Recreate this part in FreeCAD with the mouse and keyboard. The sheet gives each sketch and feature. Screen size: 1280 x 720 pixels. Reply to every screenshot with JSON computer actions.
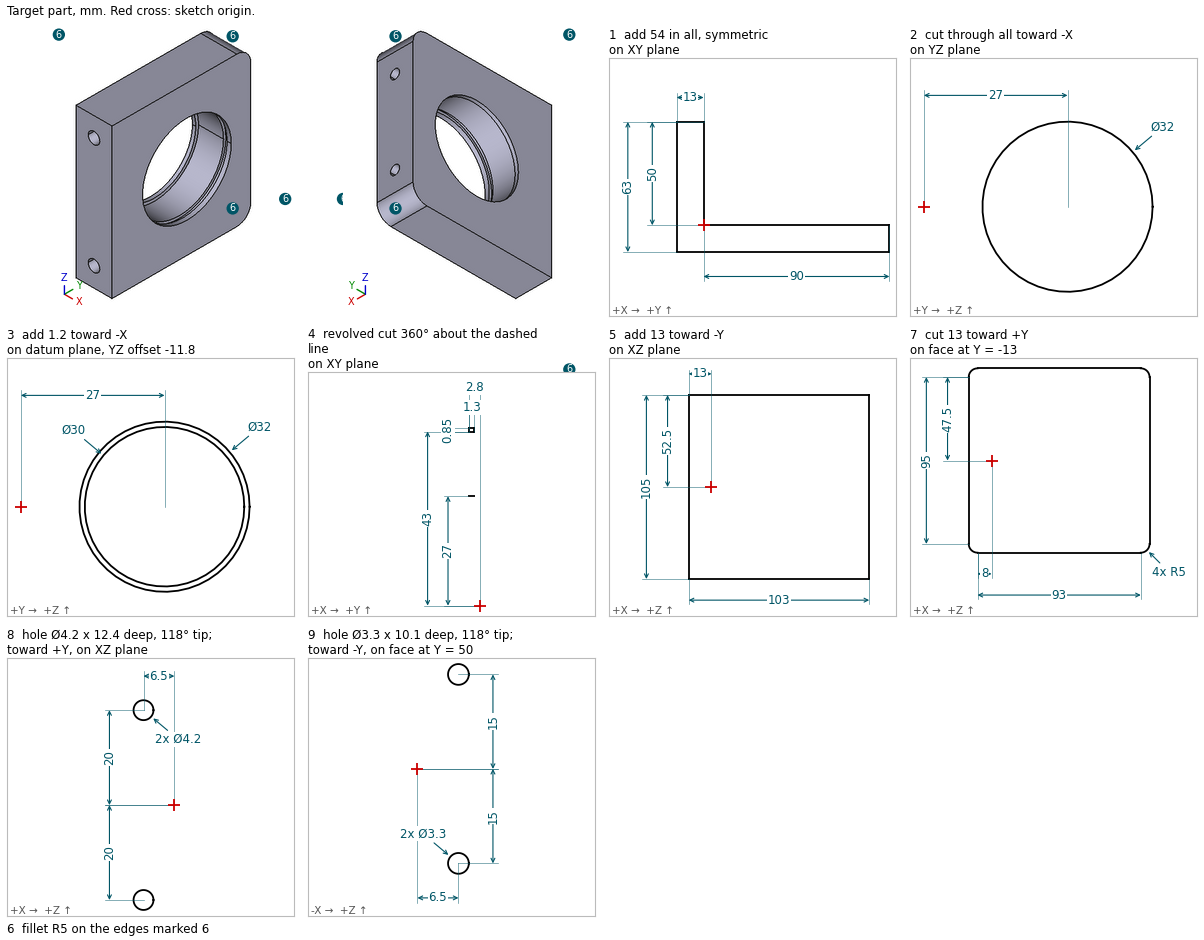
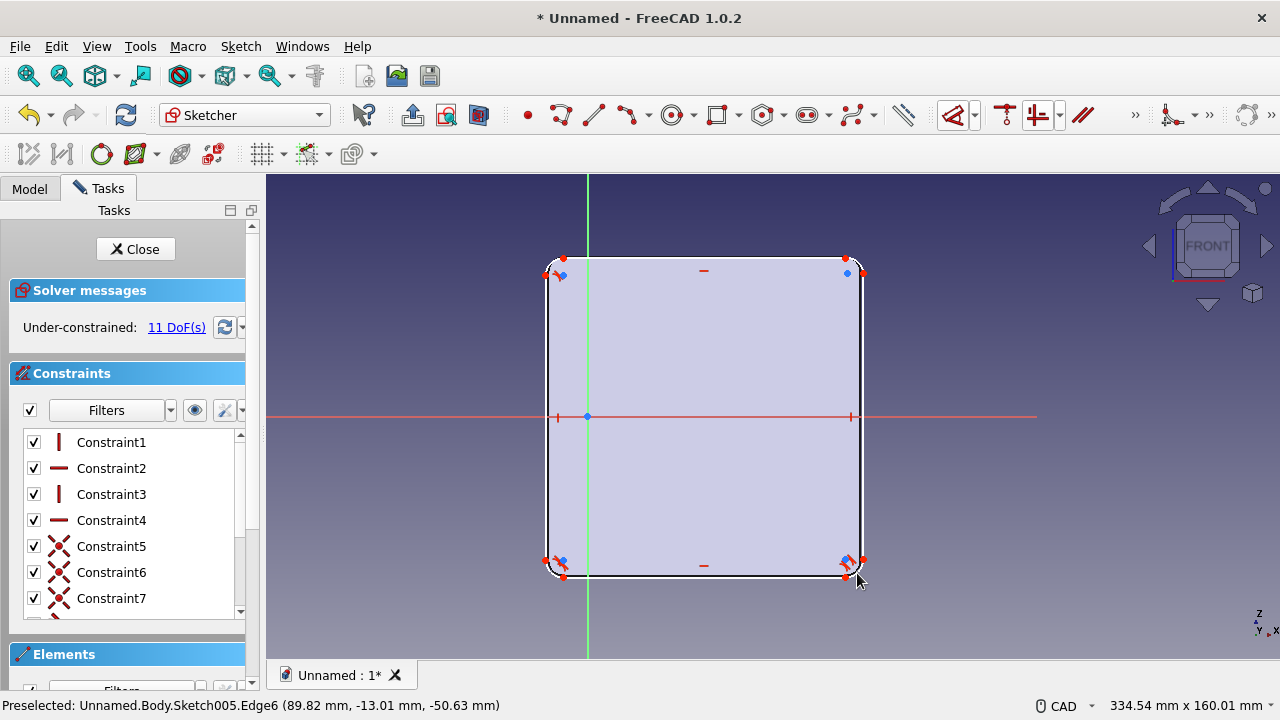
{"action": "left_click", "coordinate": [863, 474]}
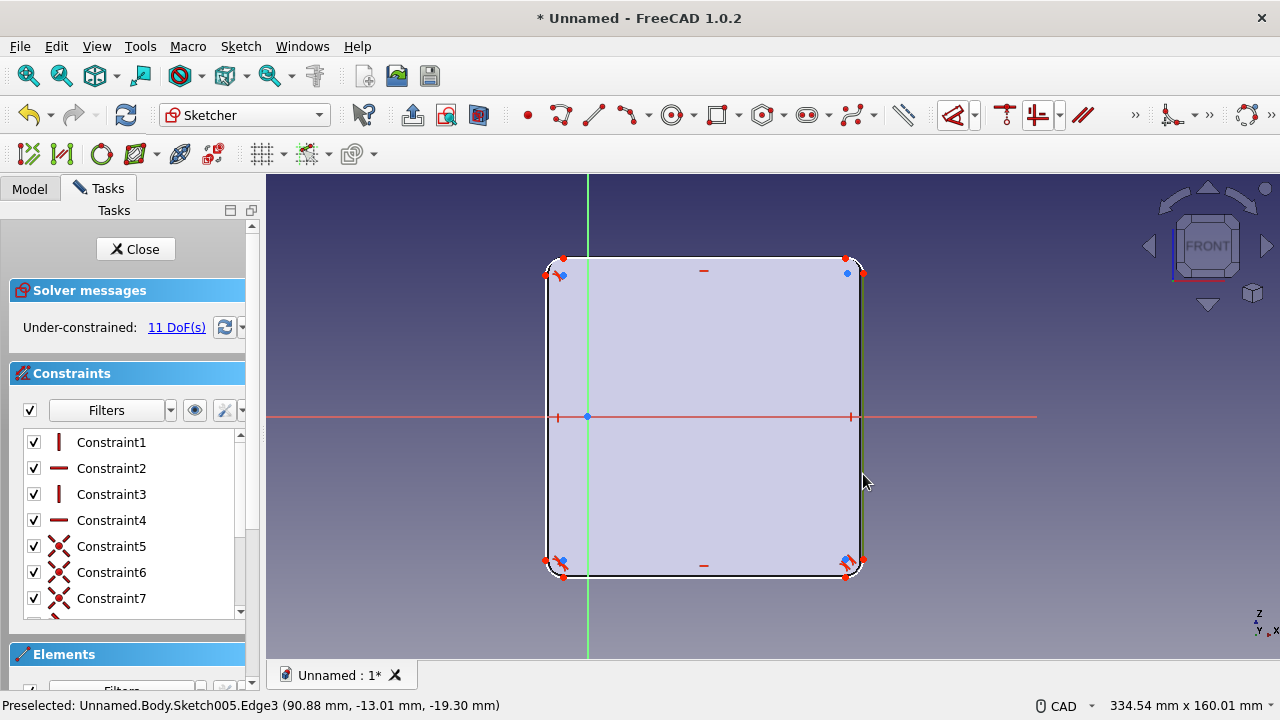
{"action": "left_click", "coordinate": [858, 262]}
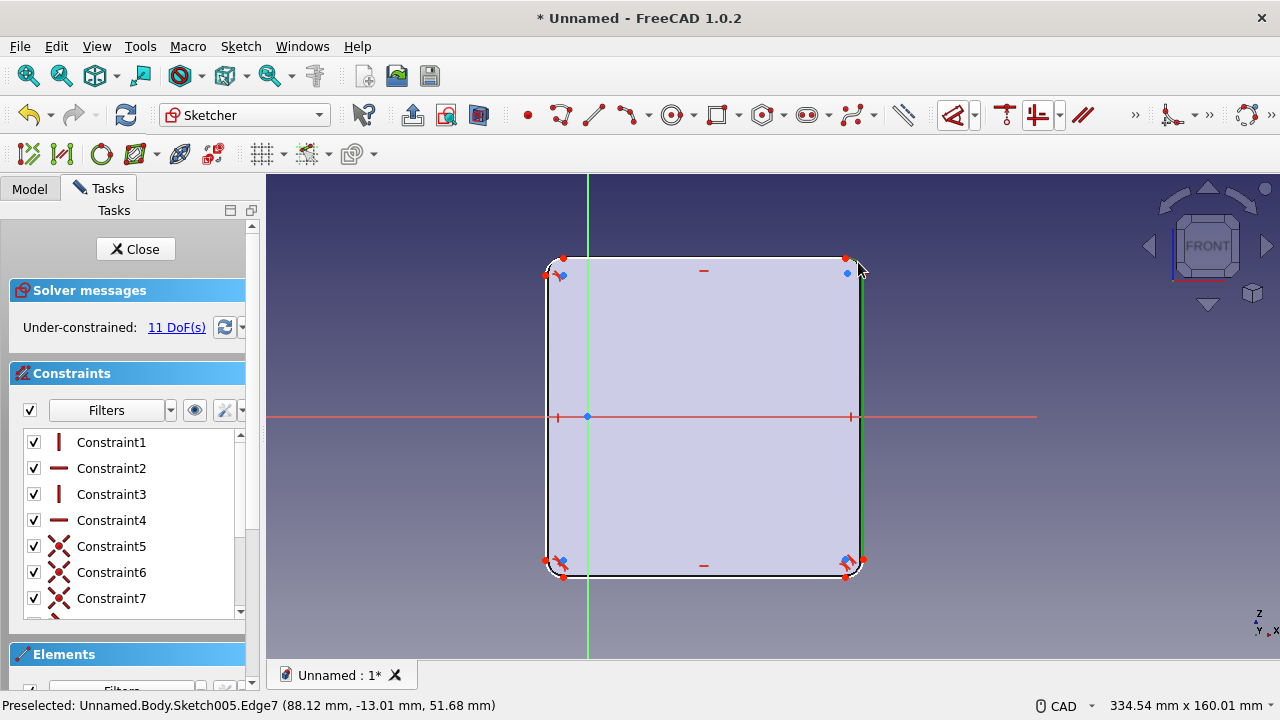
{"action": "key", "text": "t"}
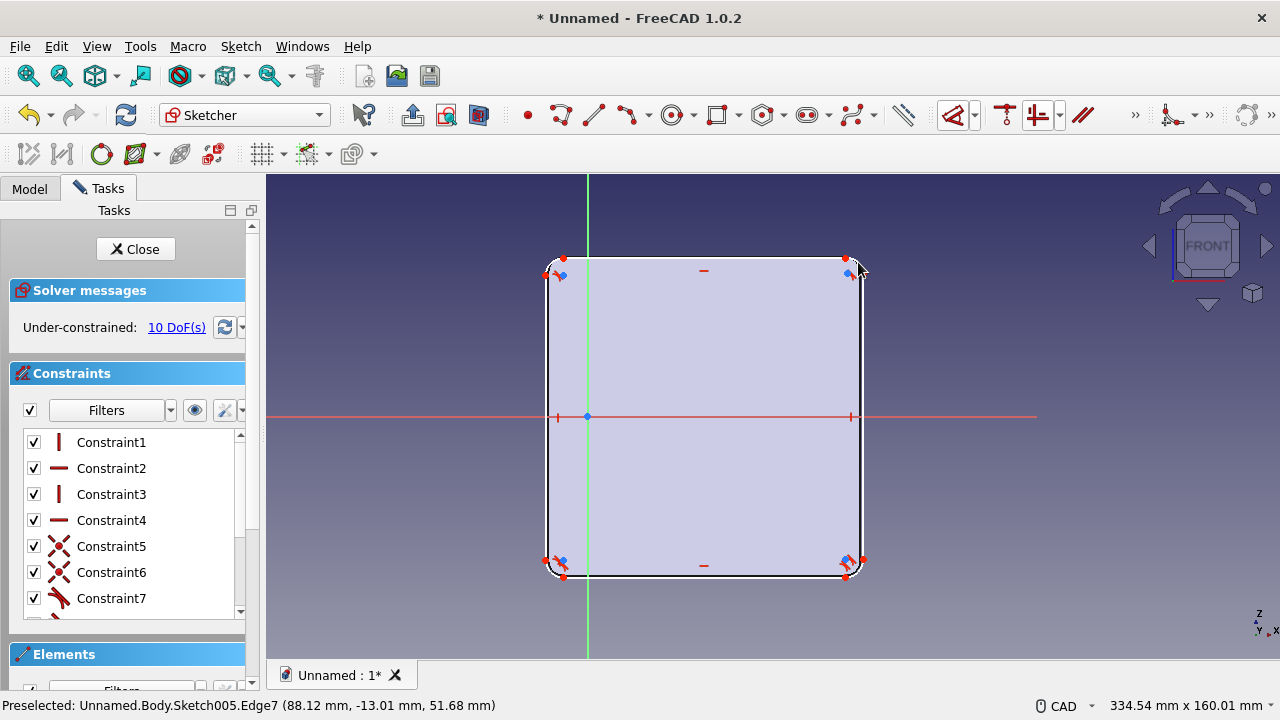
{"action": "left_click", "coordinate": [761, 258]}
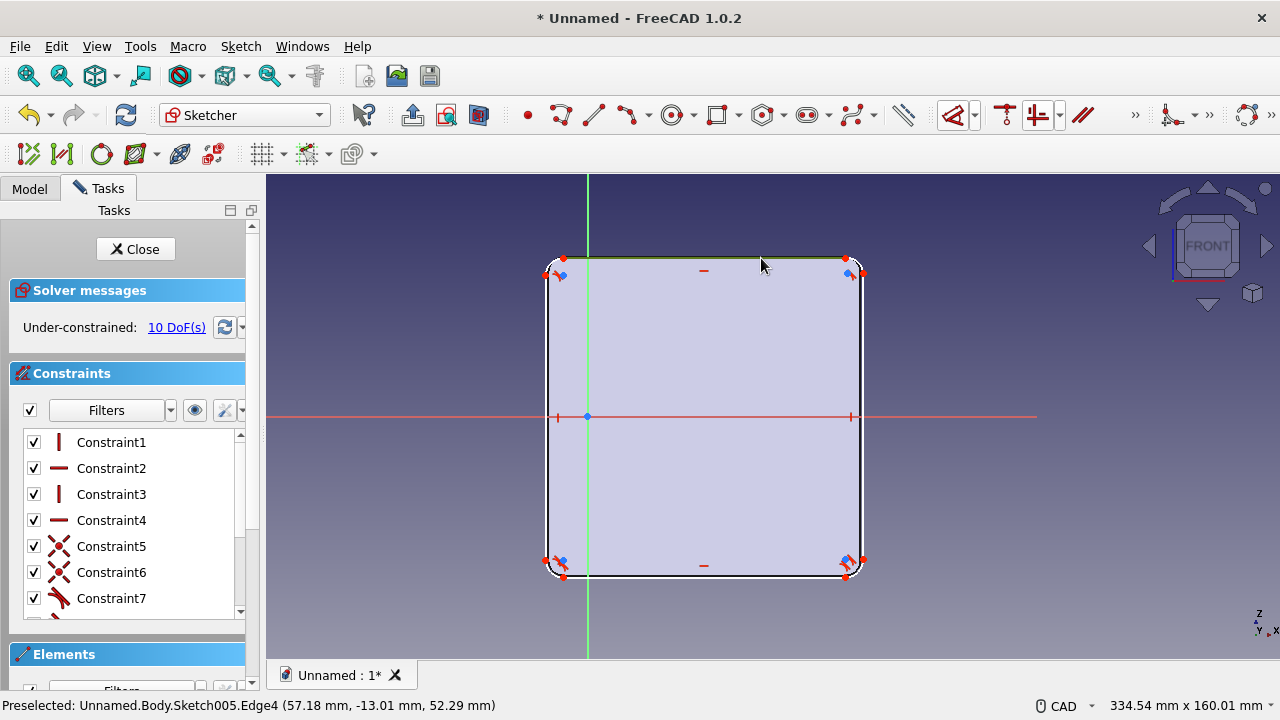
{"action": "left_click", "coordinate": [858, 262]}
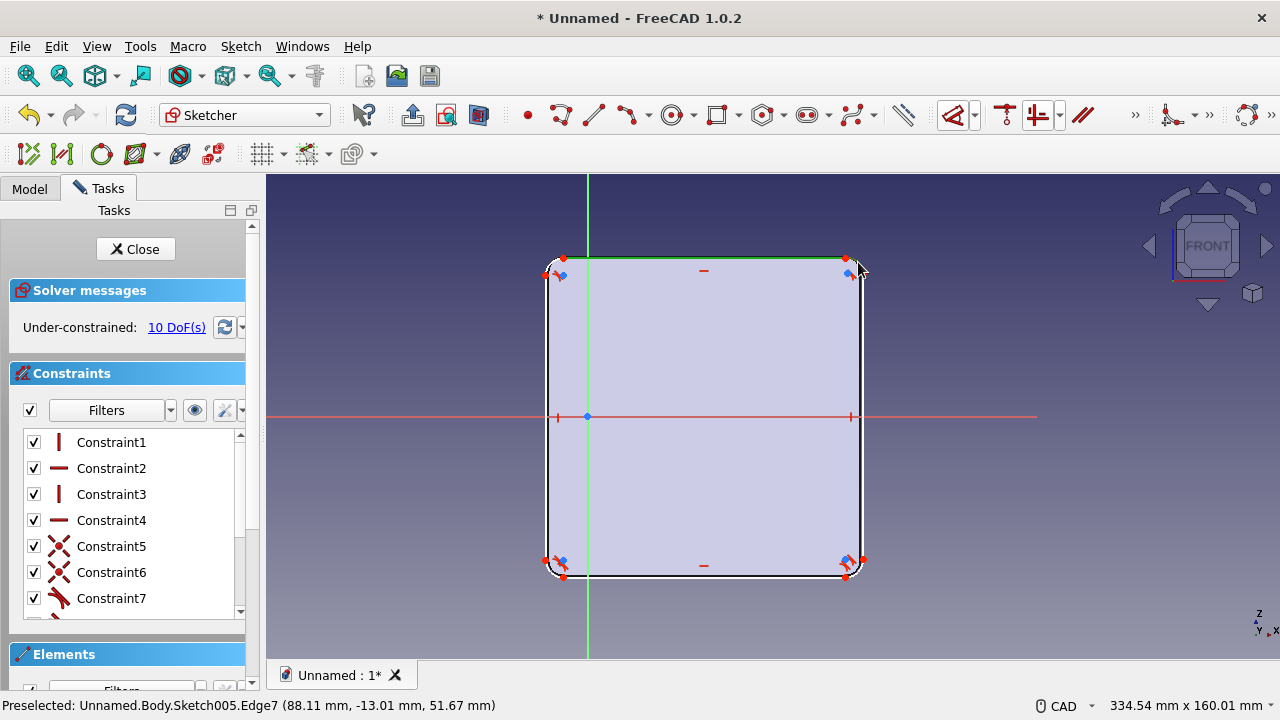
{"action": "key", "text": "t"}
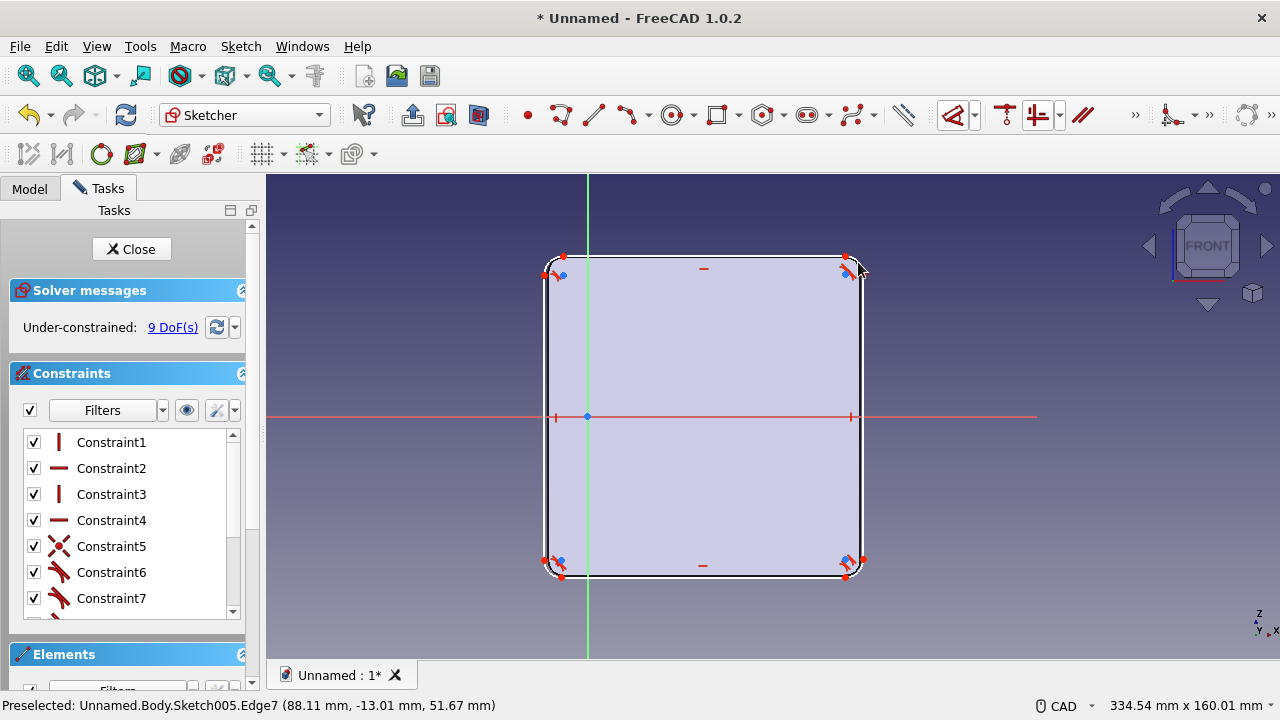
{"action": "left_click", "coordinate": [761, 256]}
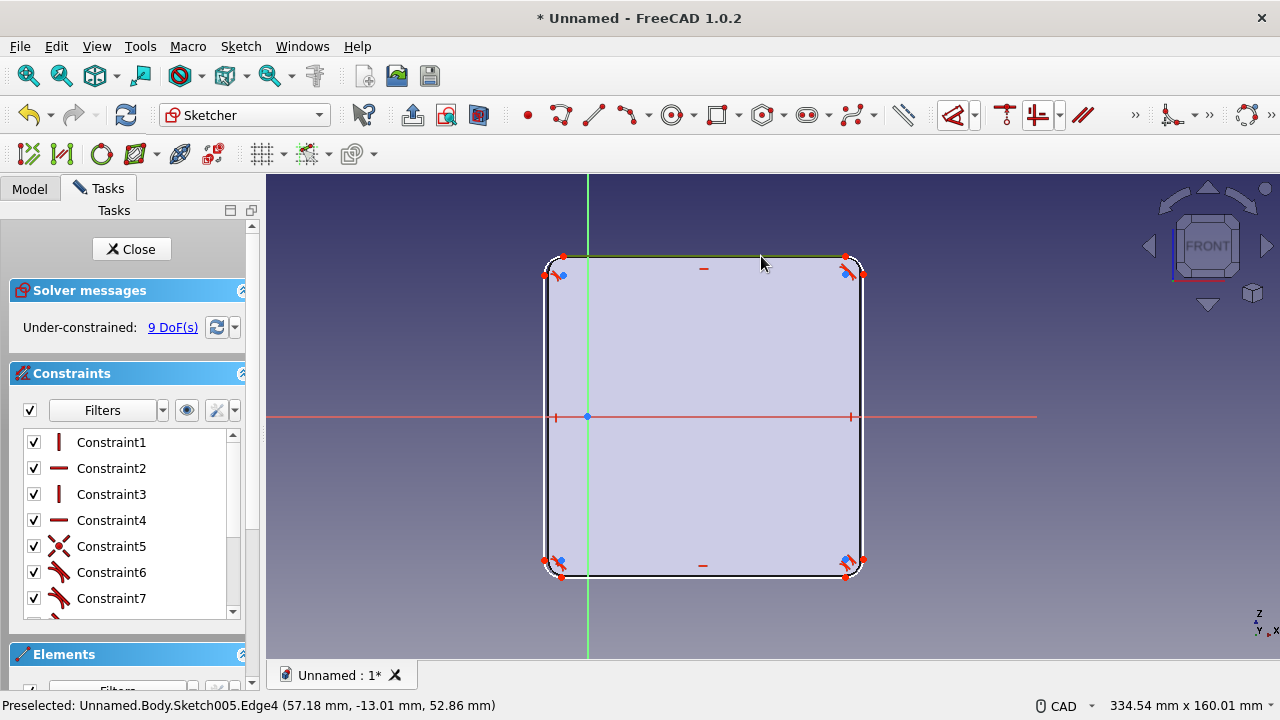
{"action": "scroll", "coordinate": [555, 258], "scroll_direction": "up", "scroll_amount": 3}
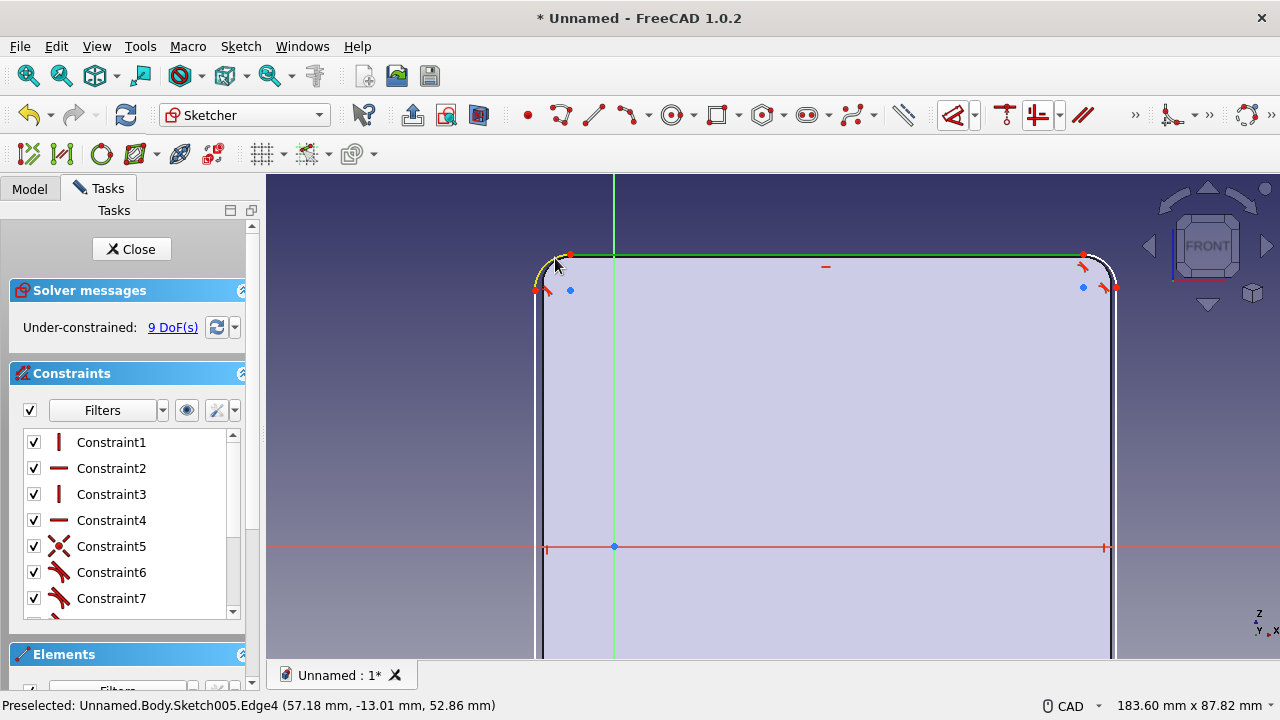
{"action": "left_click", "coordinate": [554, 259]}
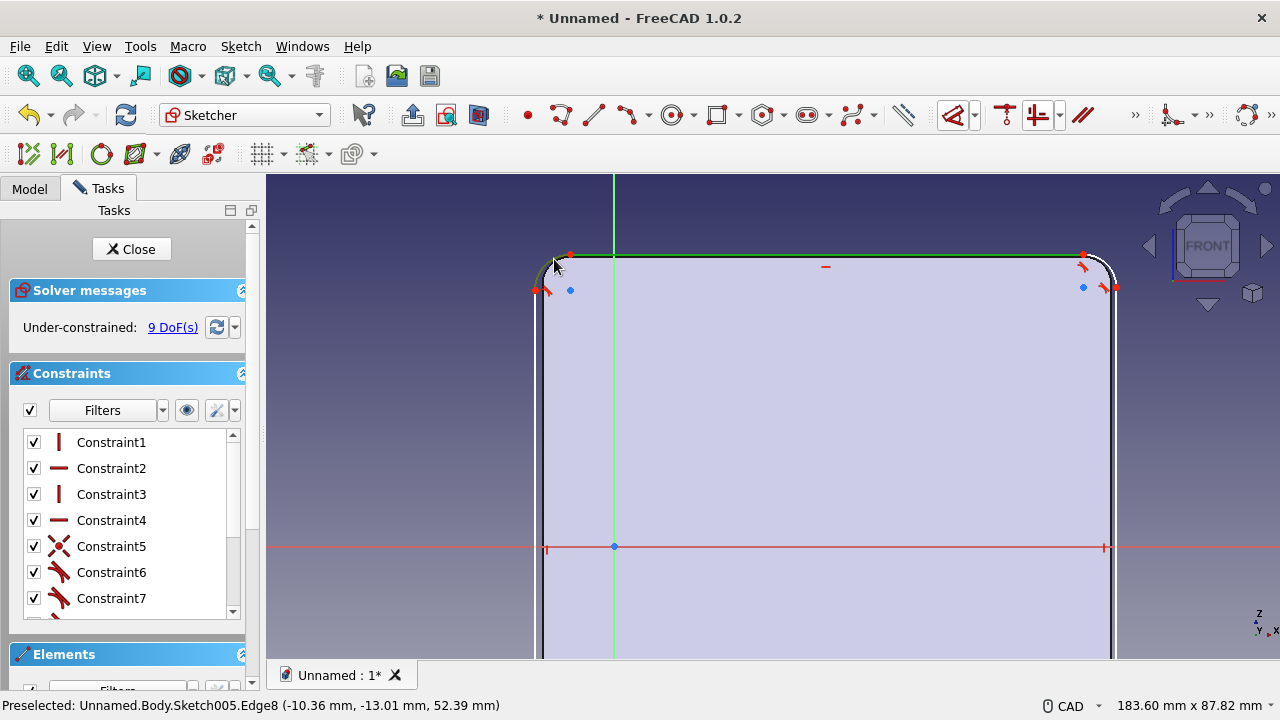
{"action": "key", "text": "t"}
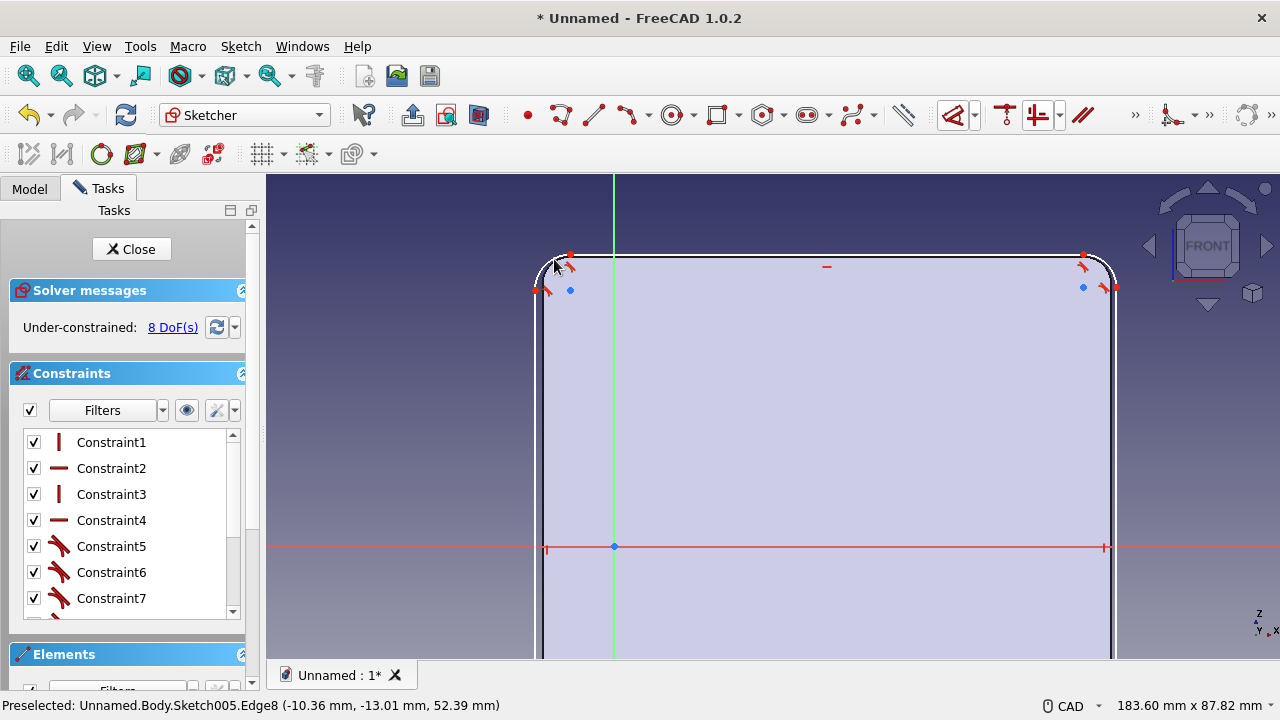
{"action": "scroll", "coordinate": [556, 258], "scroll_direction": "down", "scroll_amount": 3}